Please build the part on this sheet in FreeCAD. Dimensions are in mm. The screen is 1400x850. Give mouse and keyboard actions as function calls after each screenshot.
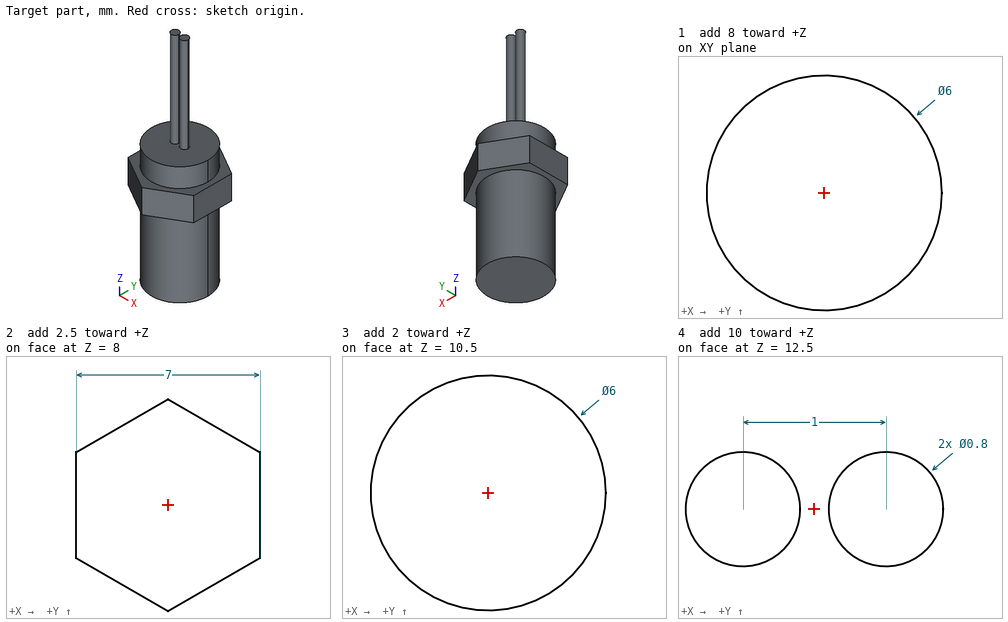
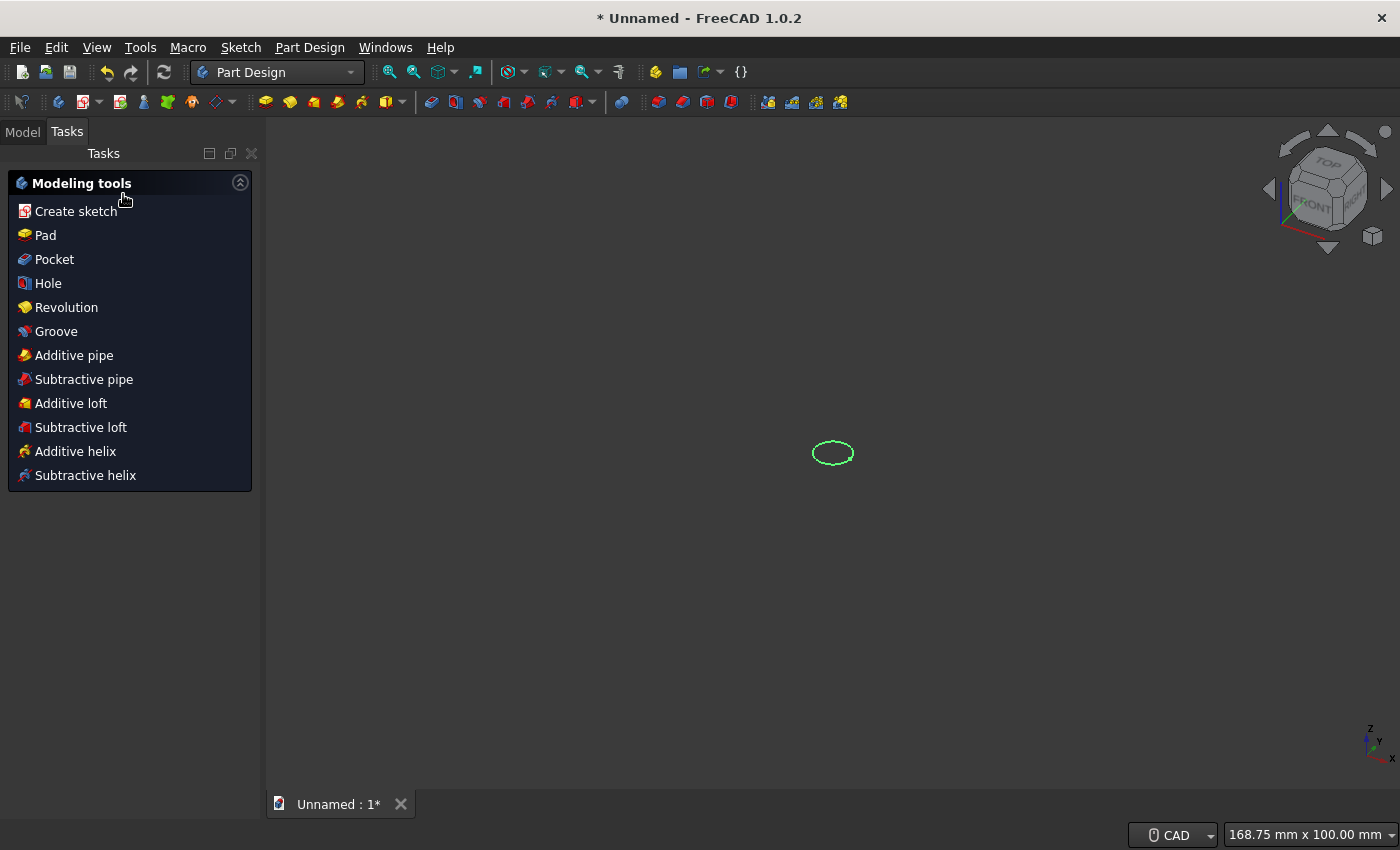
click(266, 102)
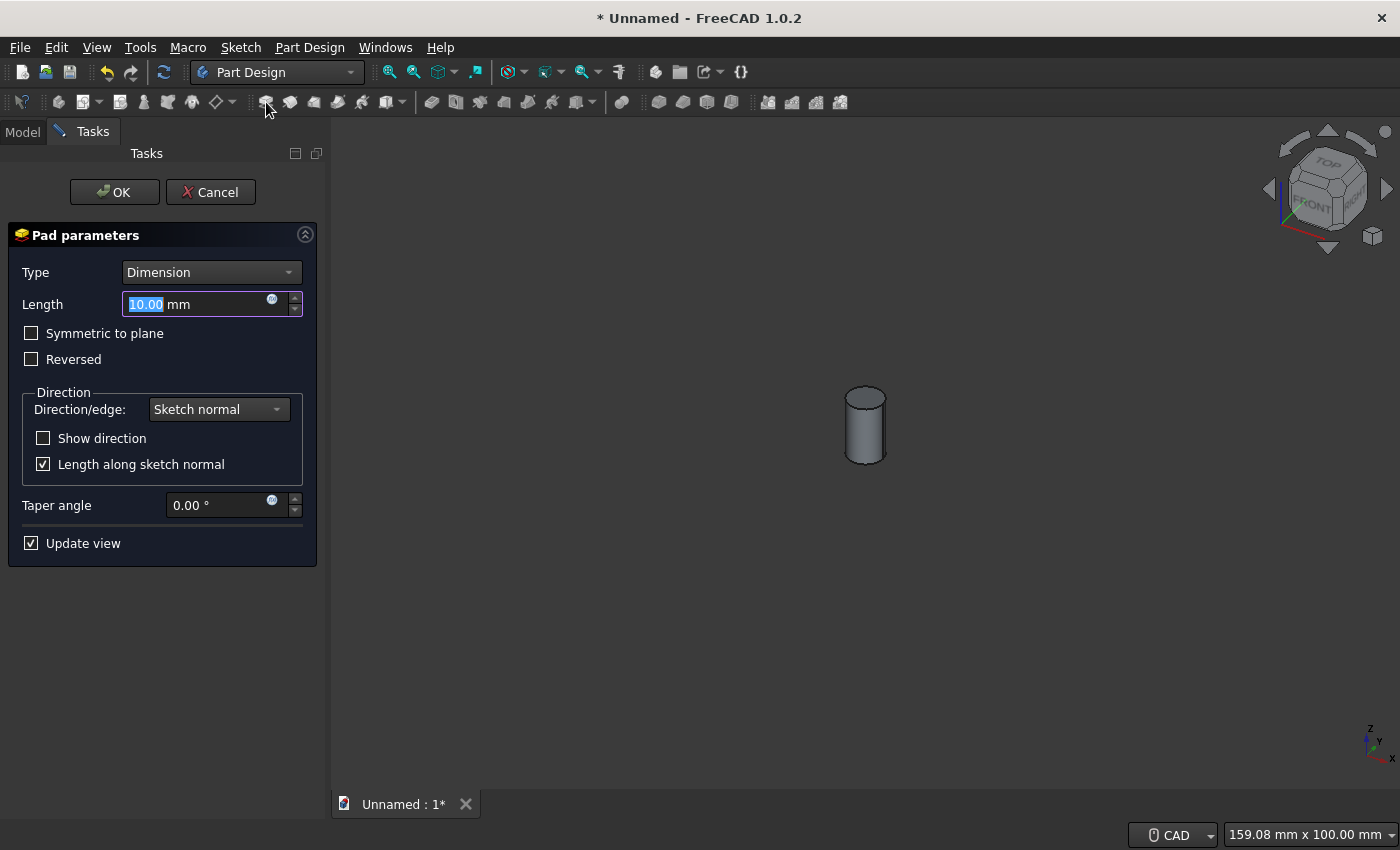
text(8)
key(Tab)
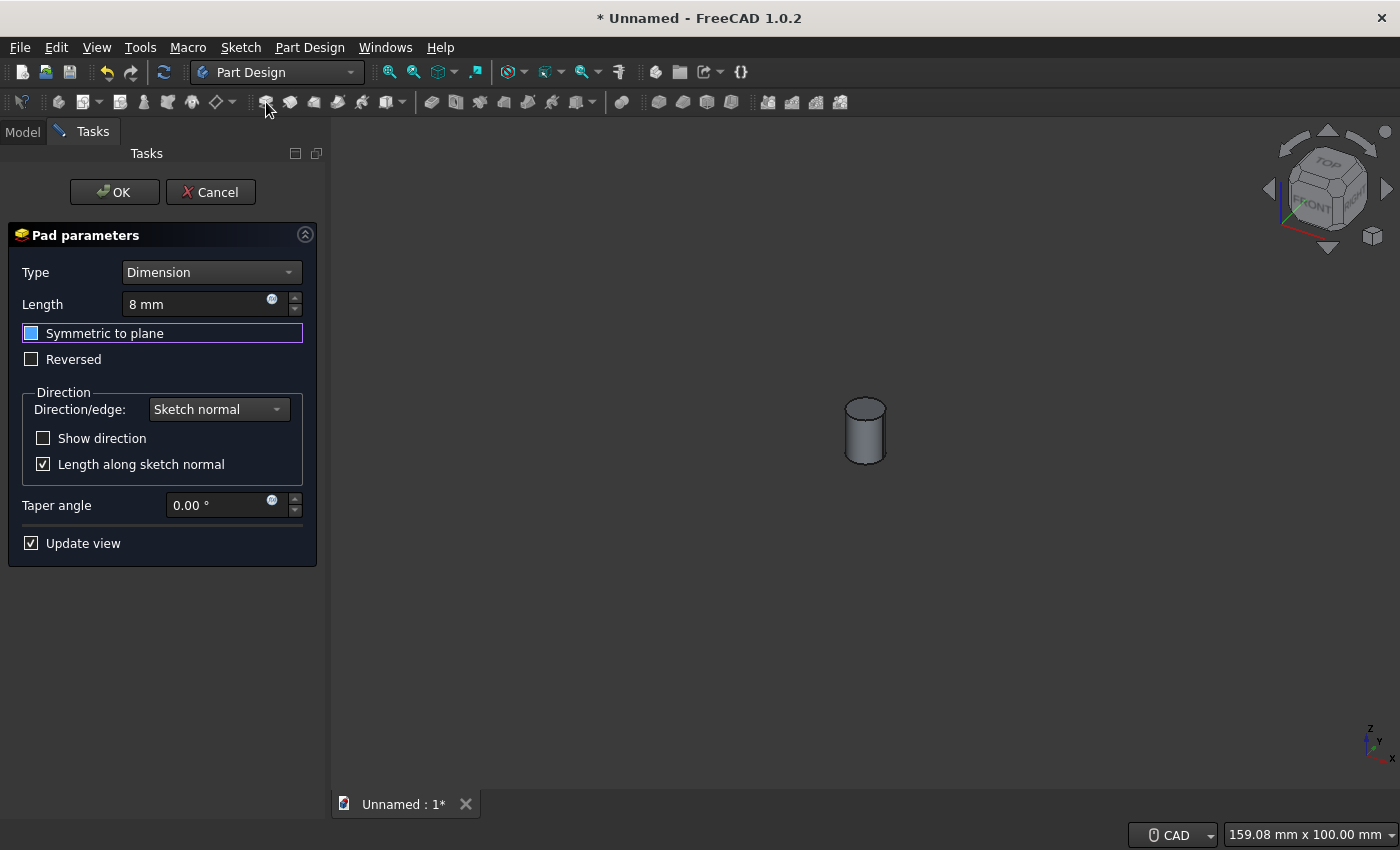
click(115, 192)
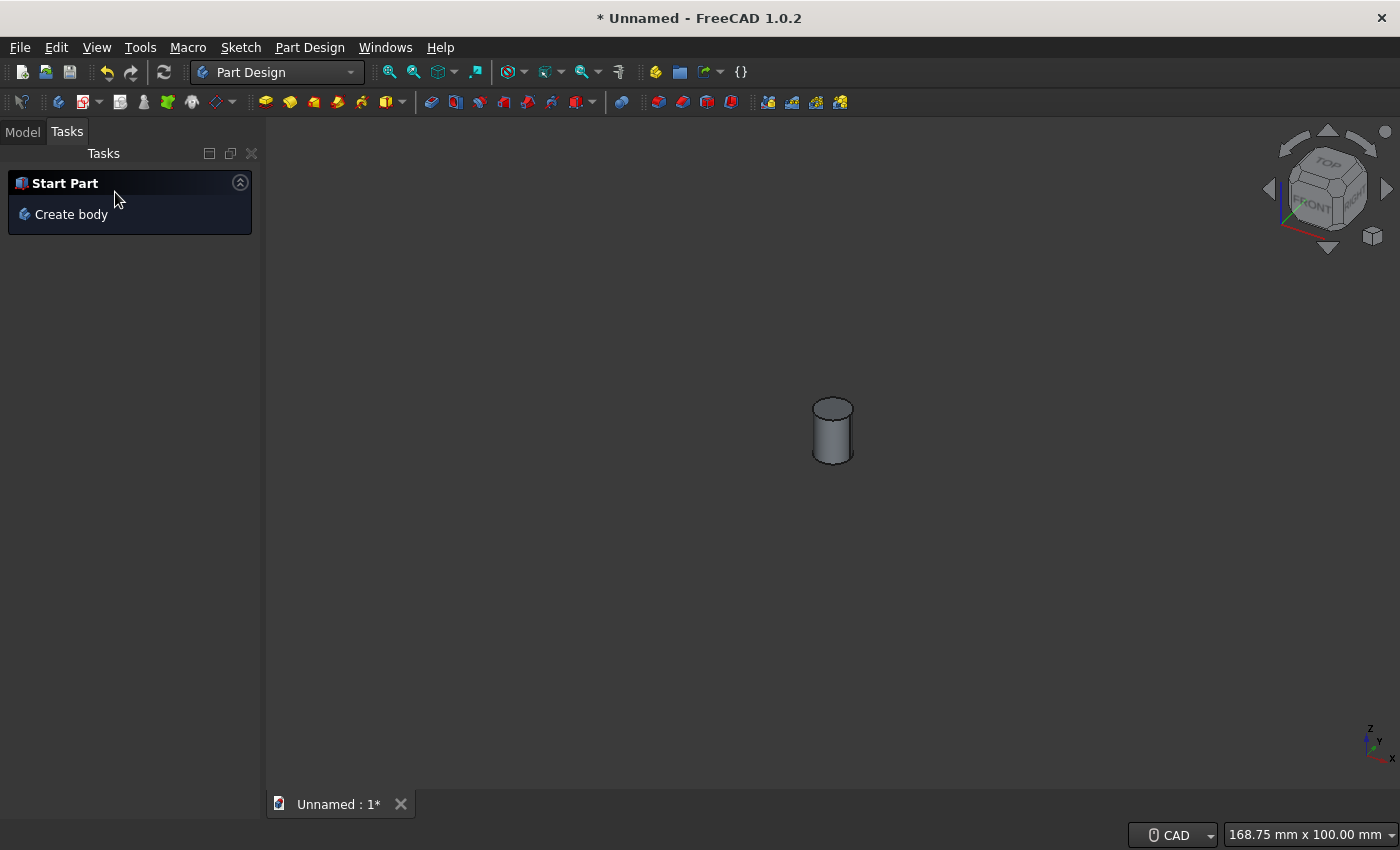
key(v)
key(f)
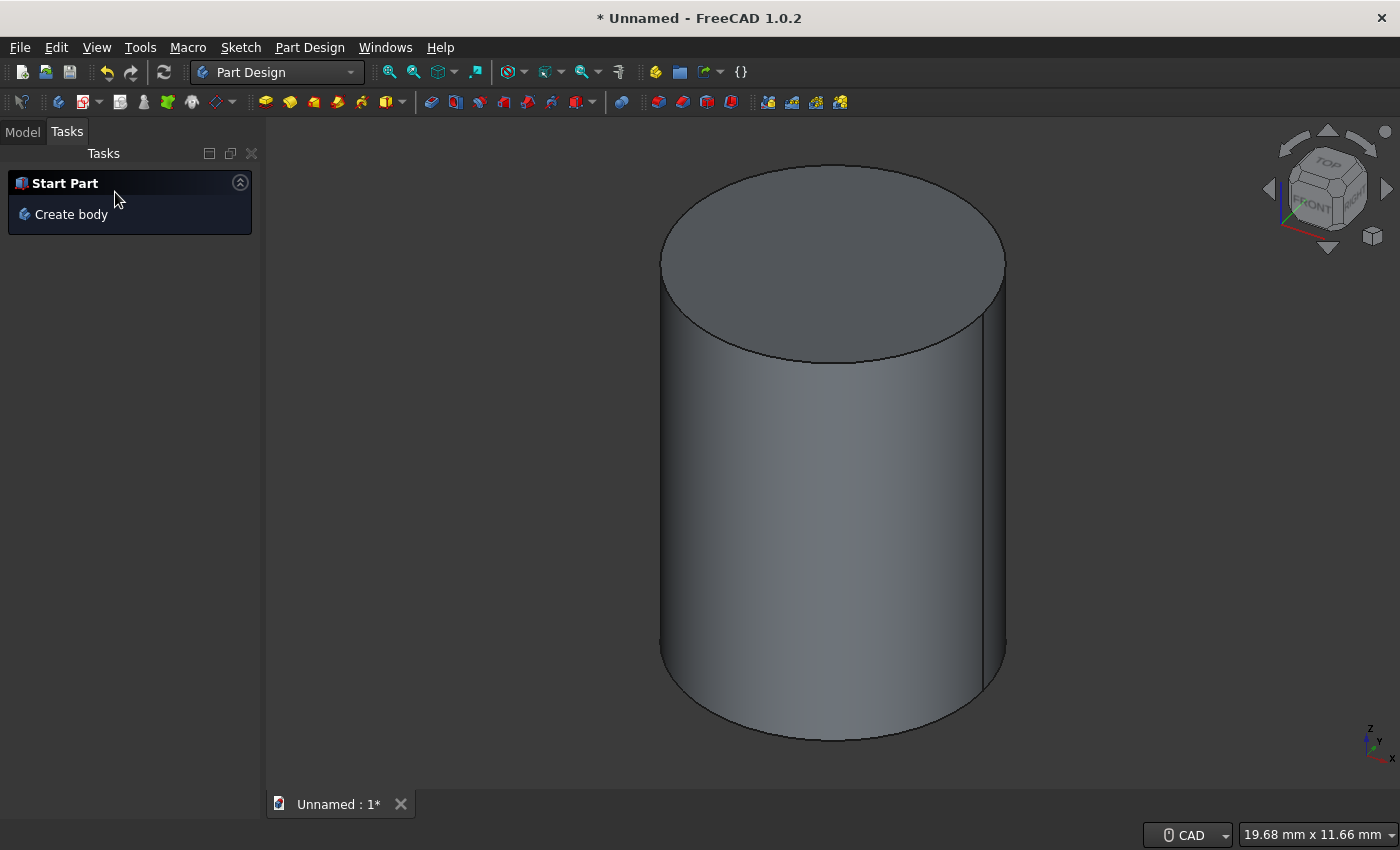
click(833, 263)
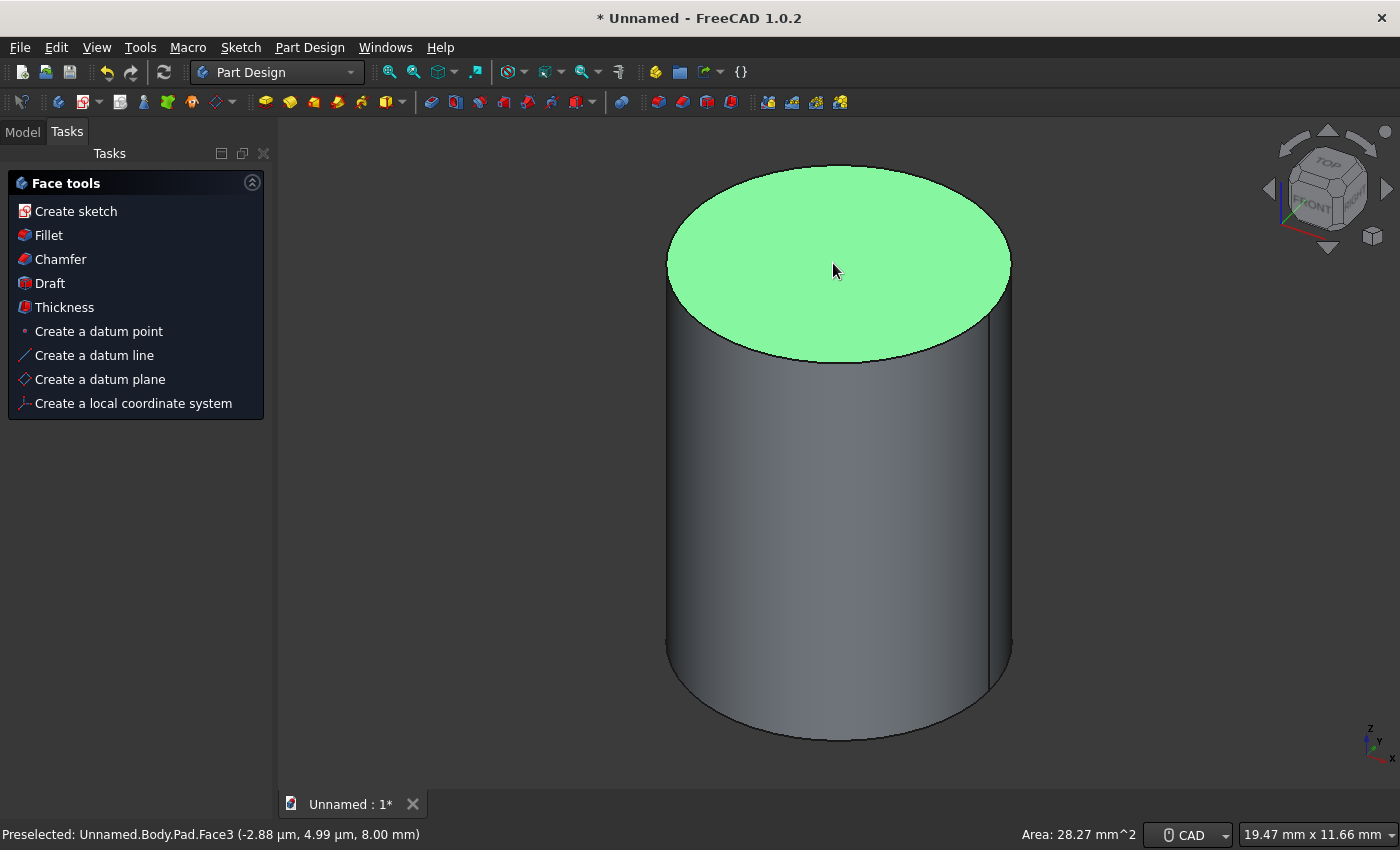
click(84, 102)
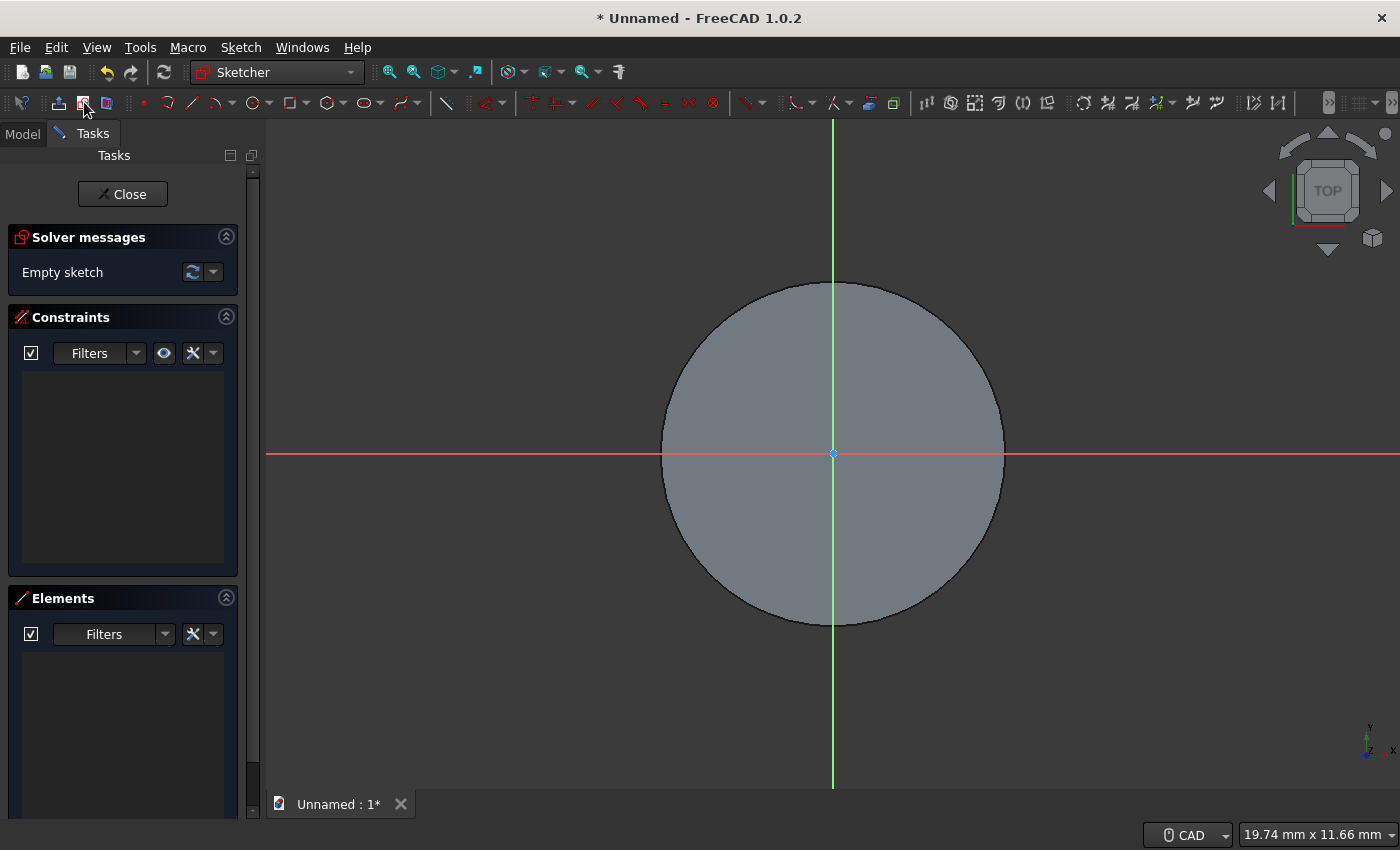
key(g)
key(p)
key(6)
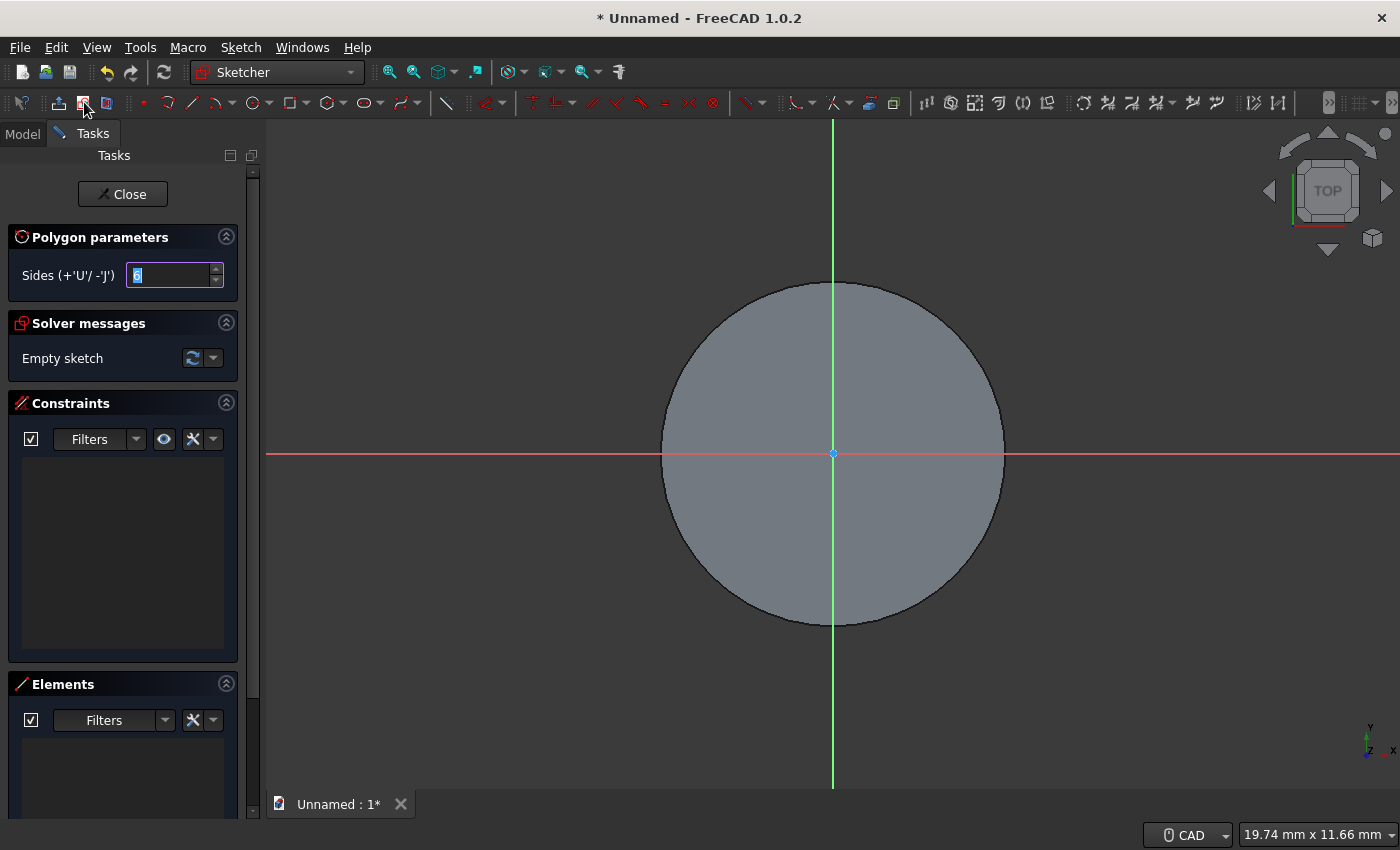
click(833, 454)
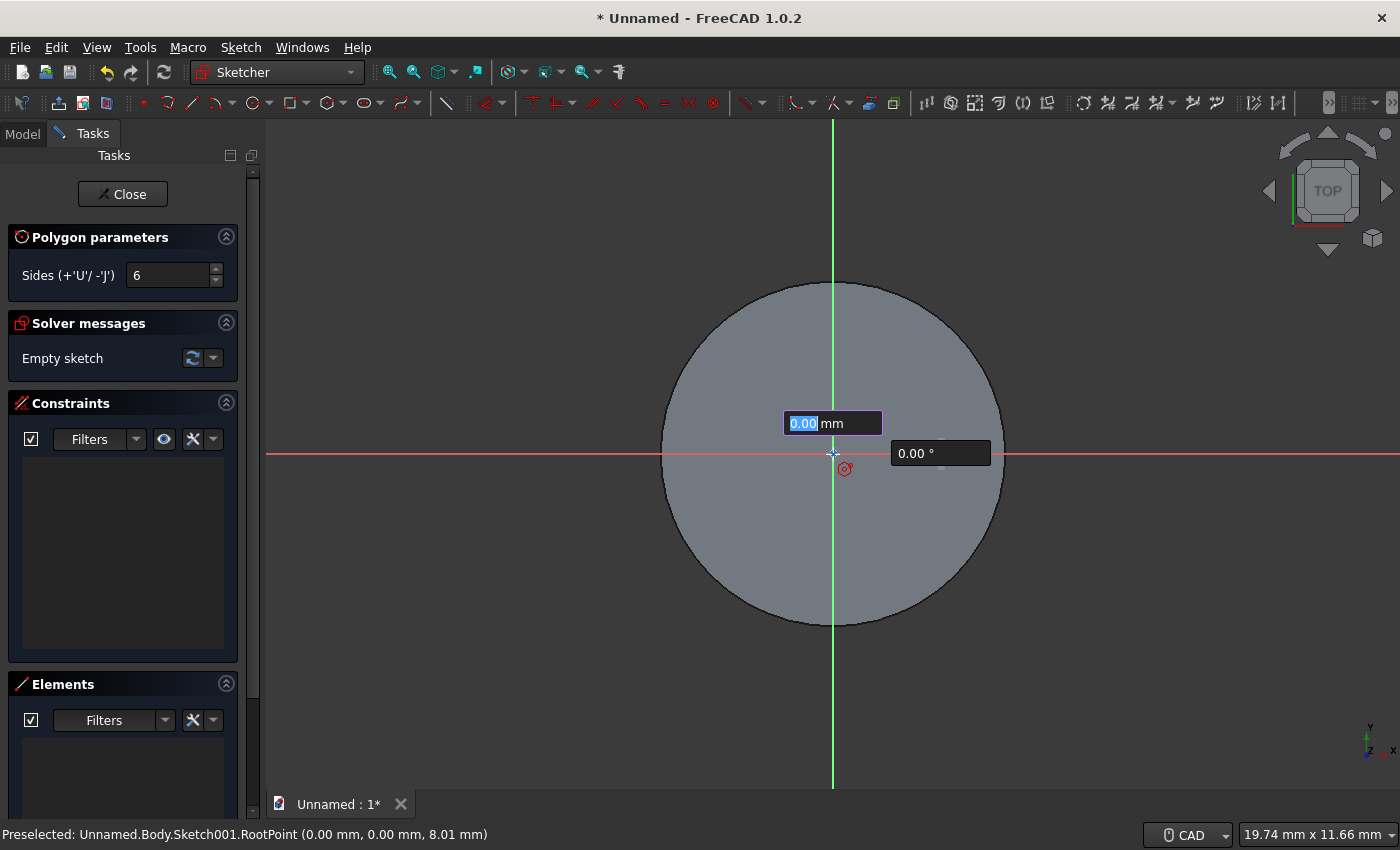
click(833, 222)
right_click(833, 222)